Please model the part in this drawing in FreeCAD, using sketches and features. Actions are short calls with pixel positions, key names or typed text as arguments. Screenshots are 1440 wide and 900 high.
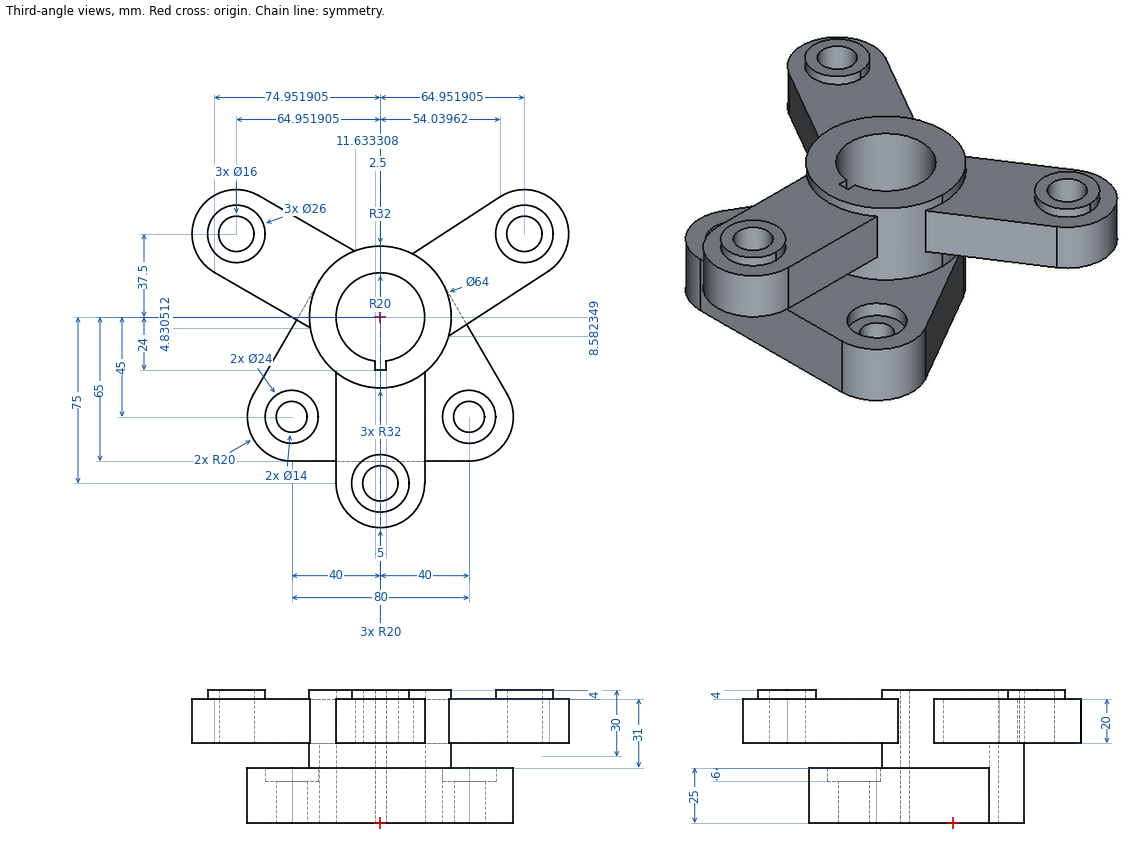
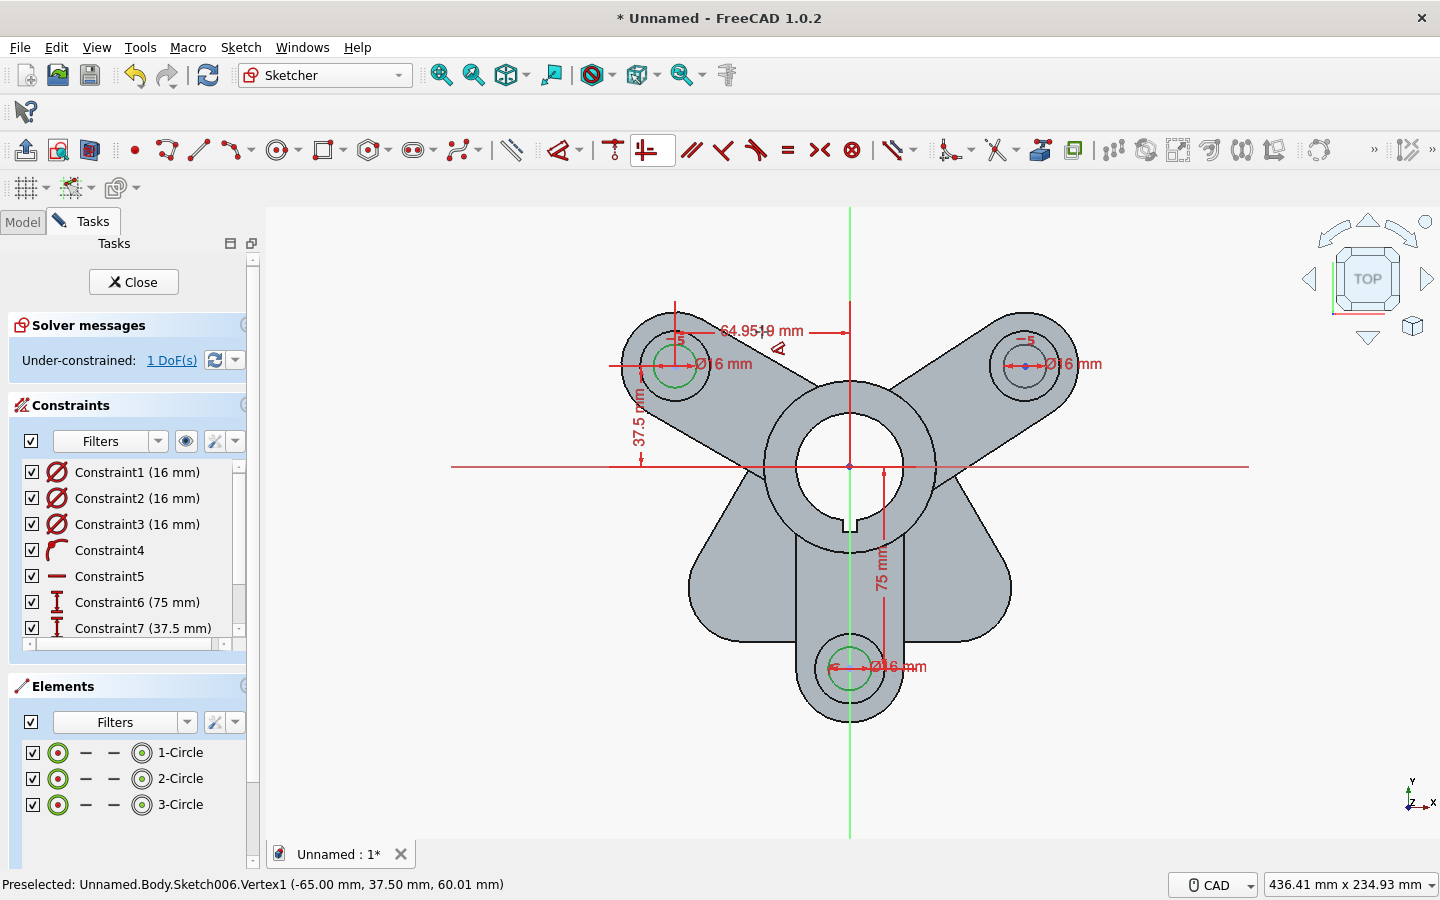
click(1025, 366)
click(937, 332)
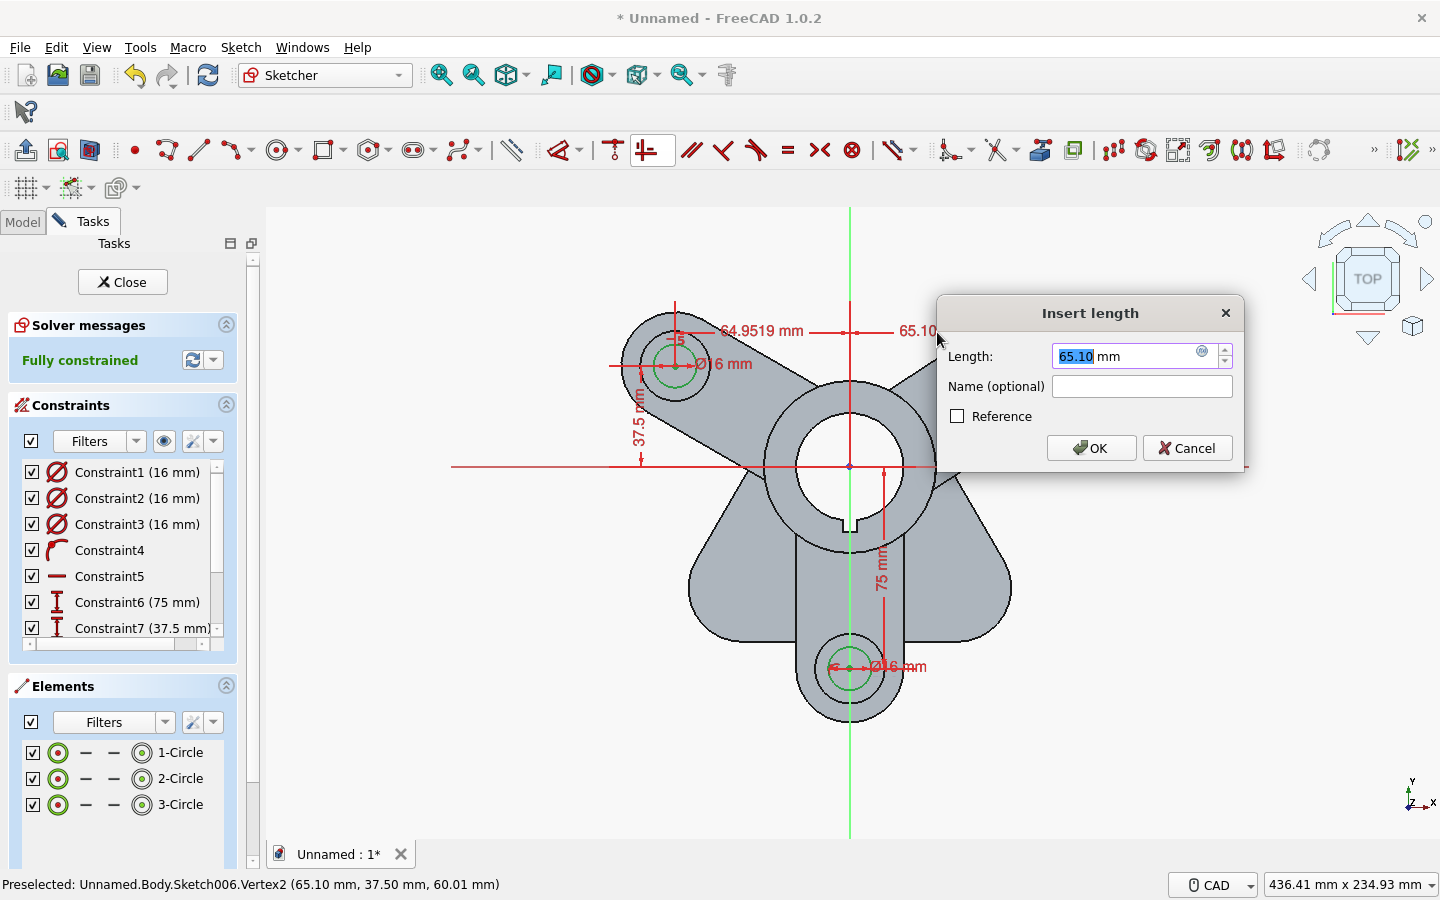
text(64.951905)
key(Return)
key(Escape)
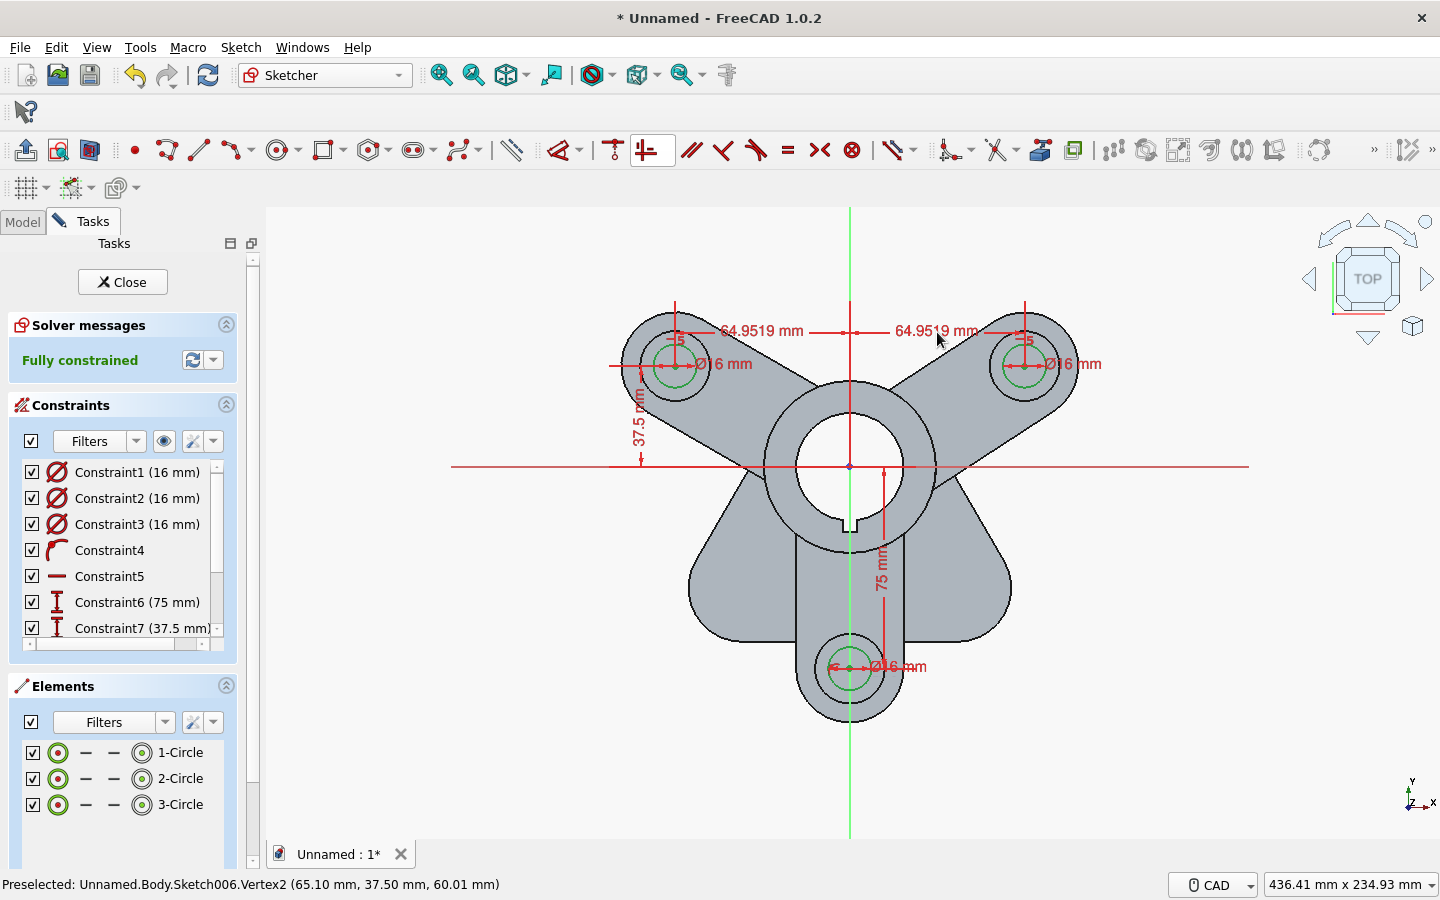
click(123, 282)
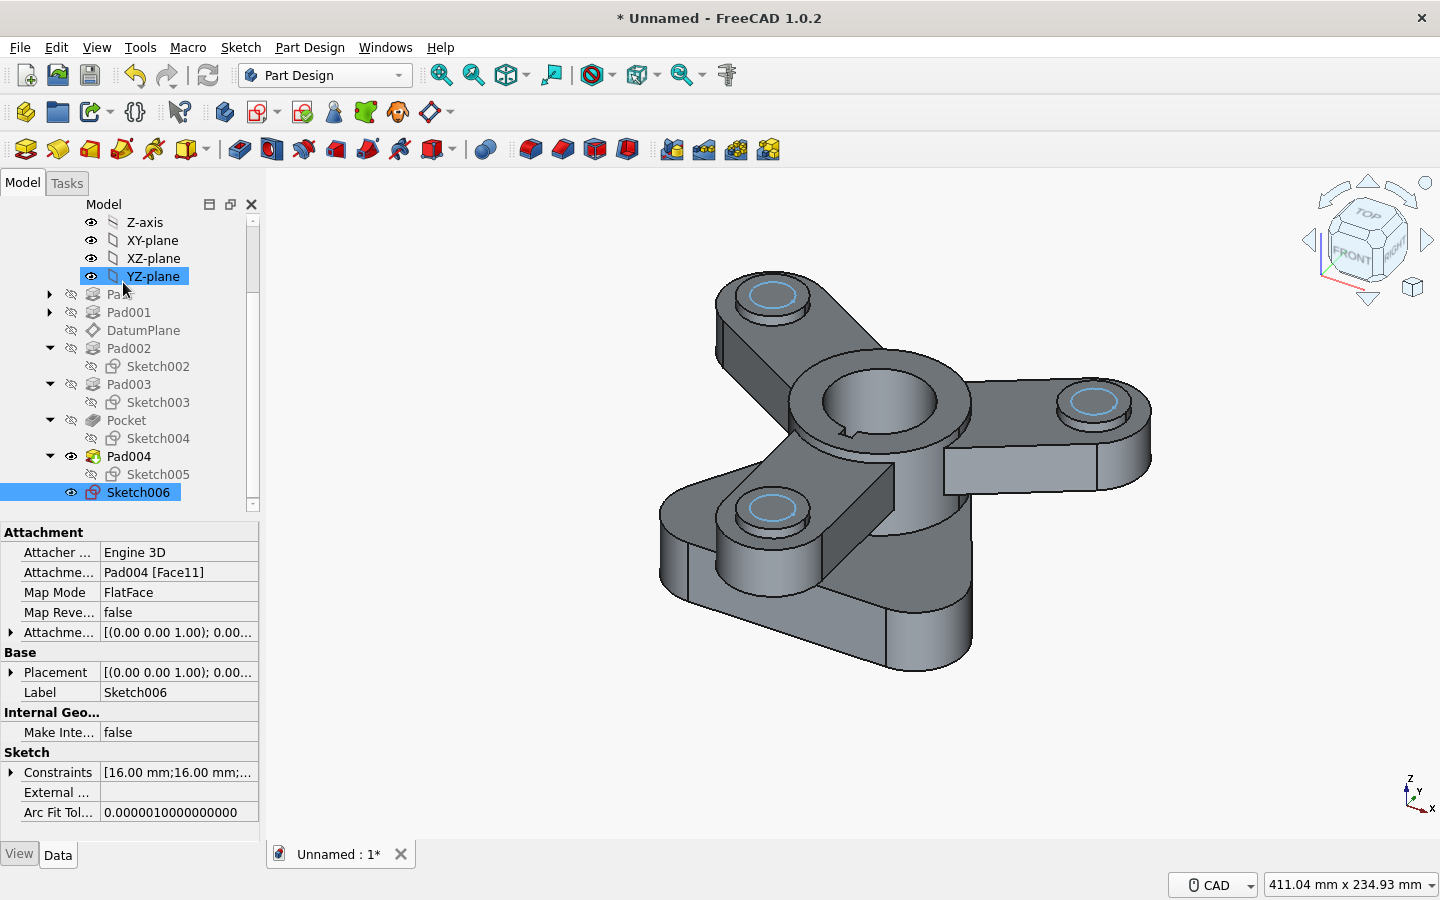
click(240, 150)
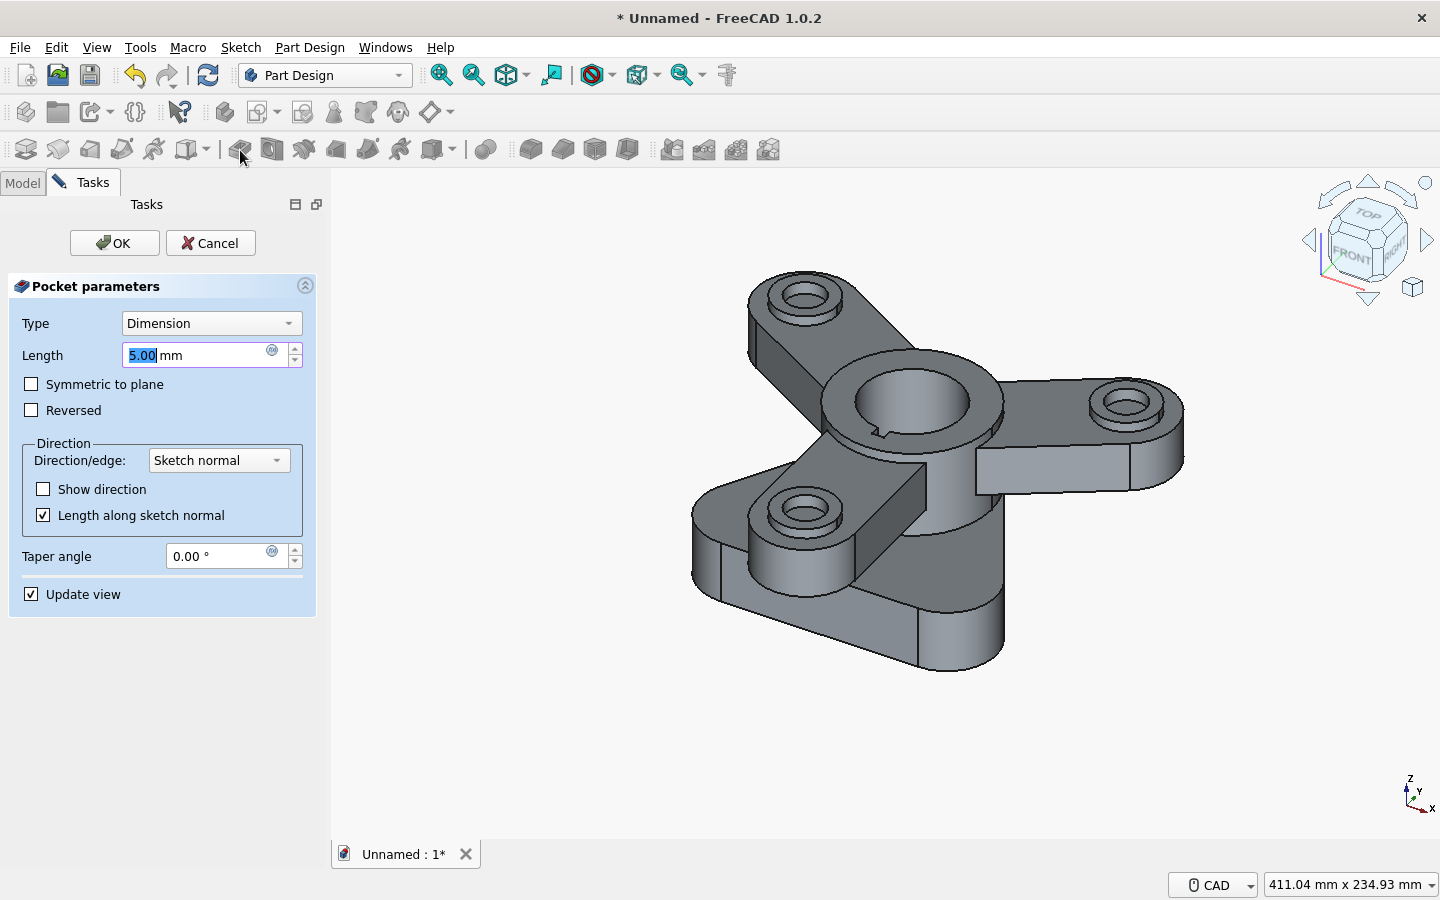
text(30)
key(Tab)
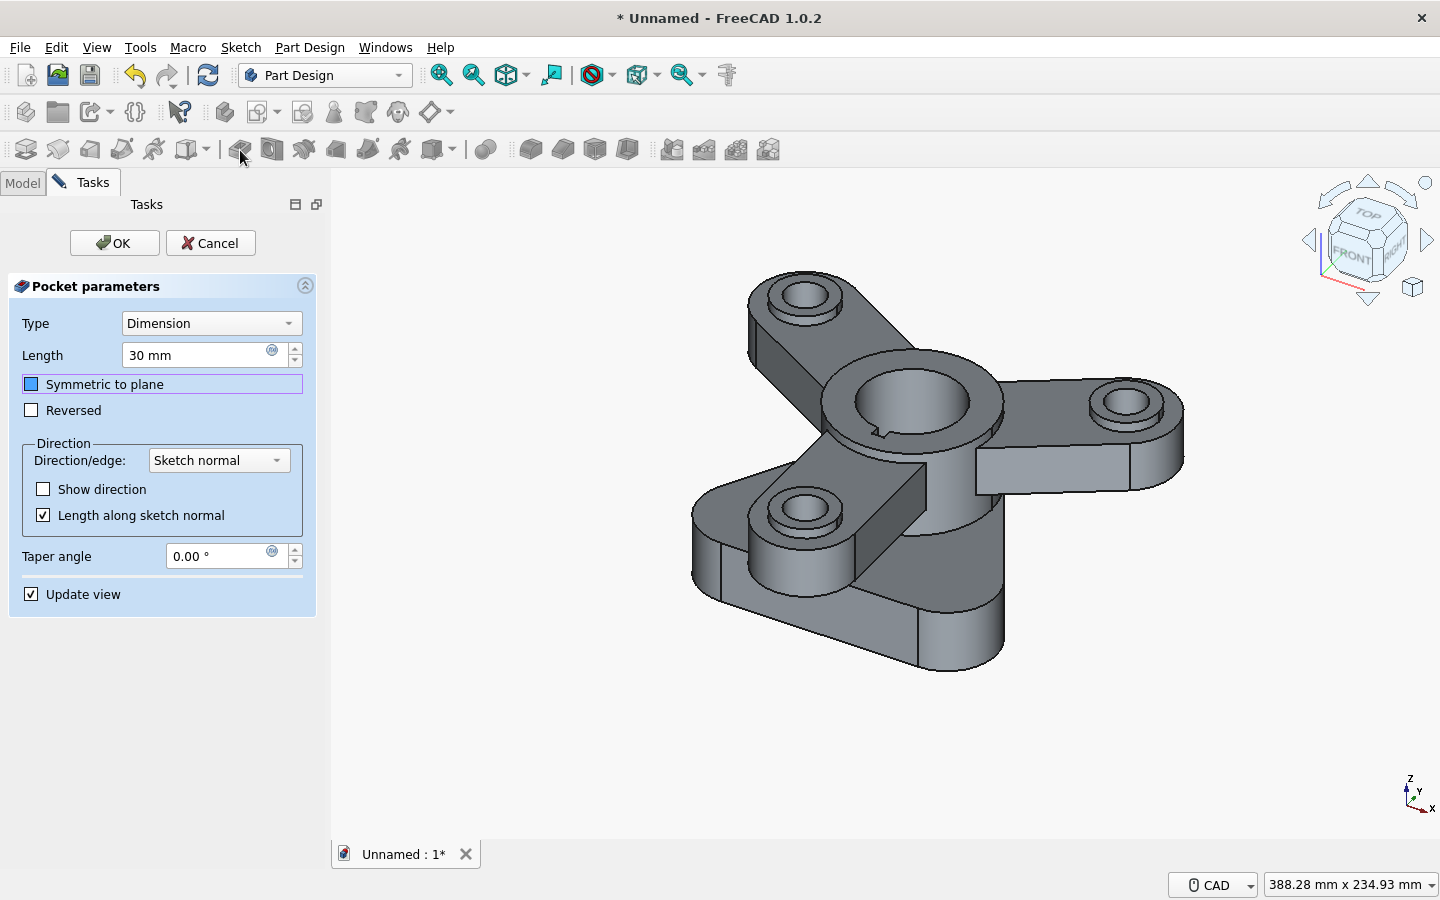
click(115, 243)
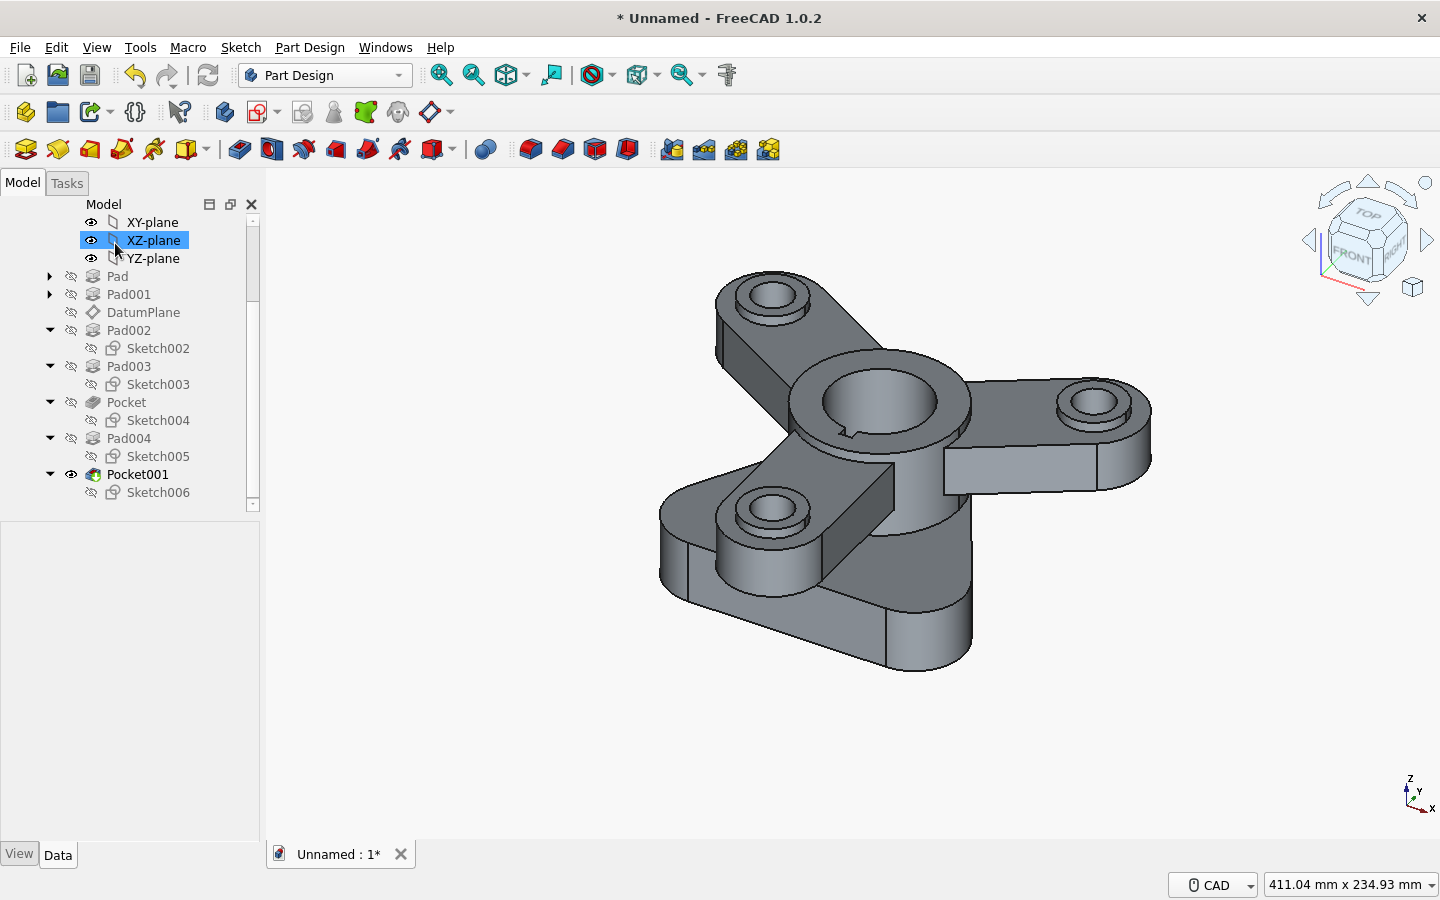
click(913, 562)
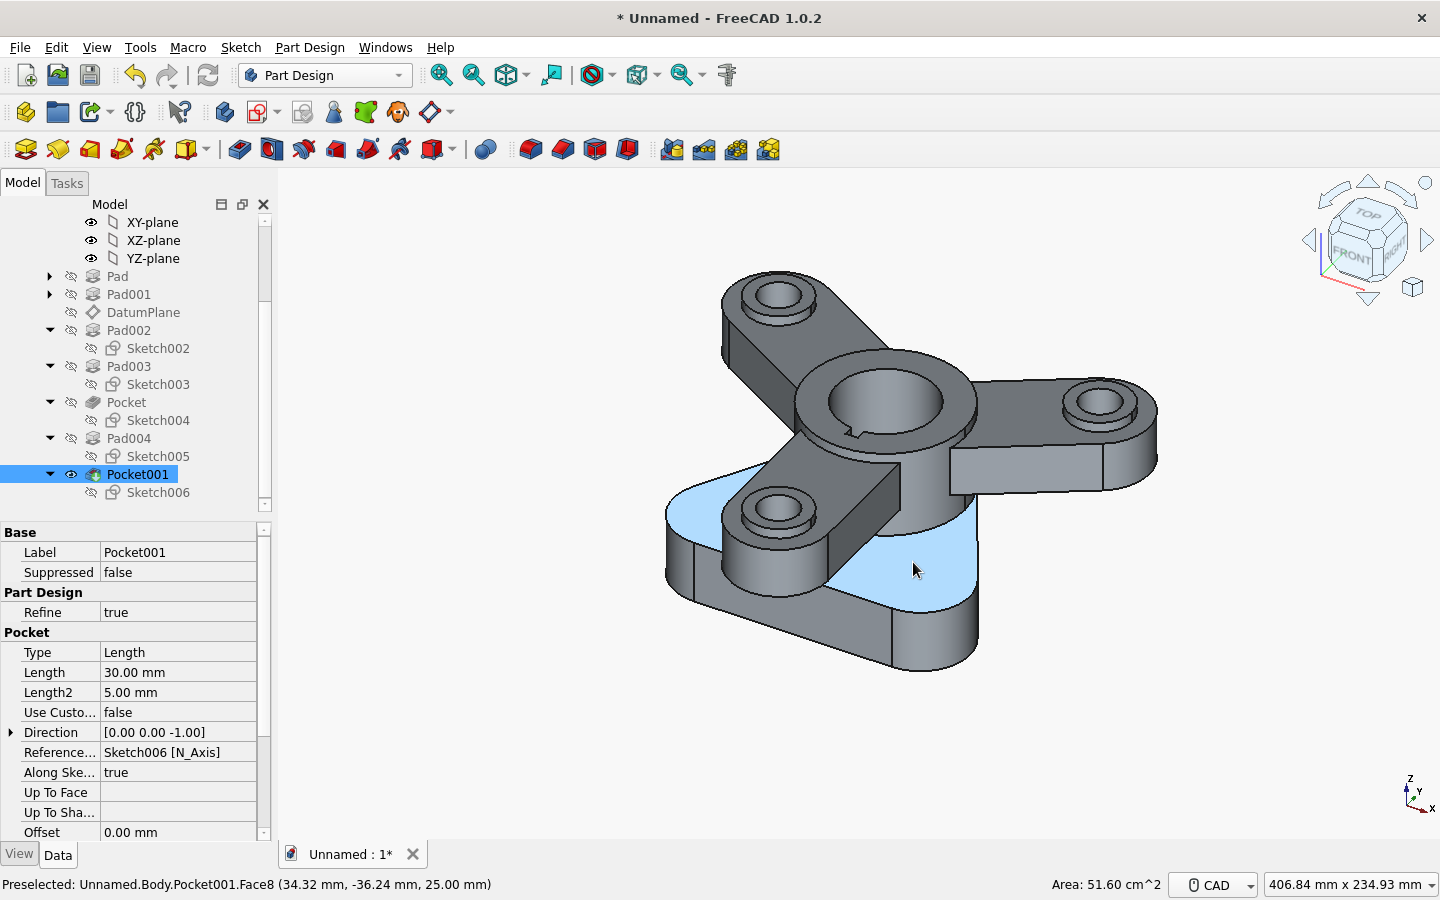
click(258, 112)